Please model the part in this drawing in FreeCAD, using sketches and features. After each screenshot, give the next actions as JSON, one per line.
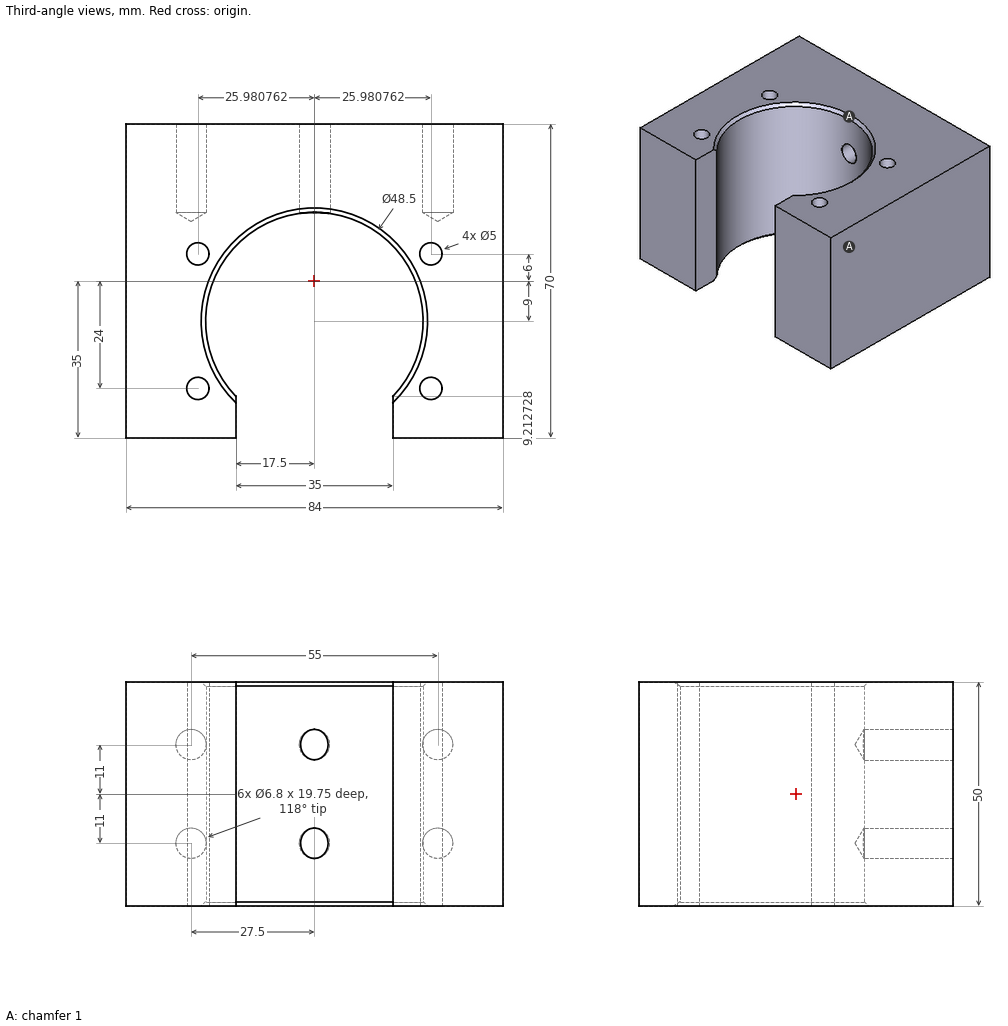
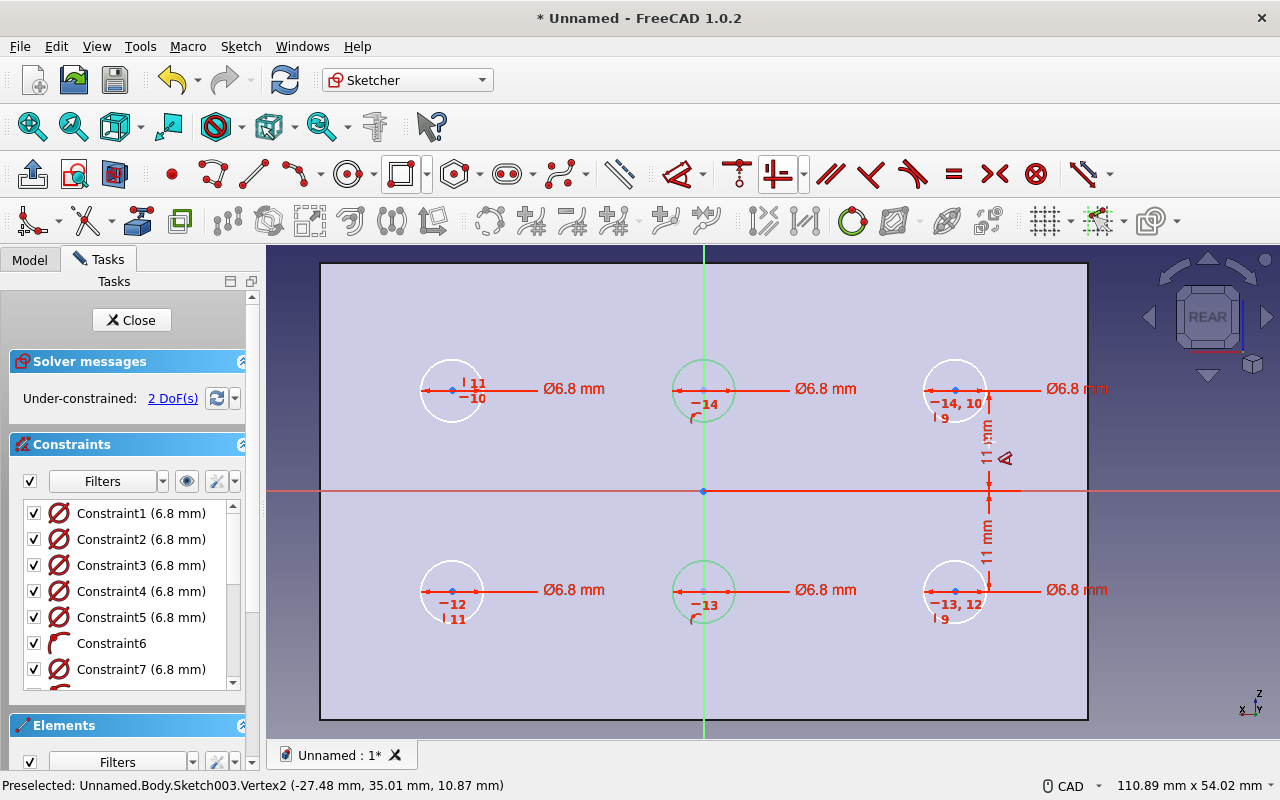
{"action": "left_click", "coordinate": [955, 391]}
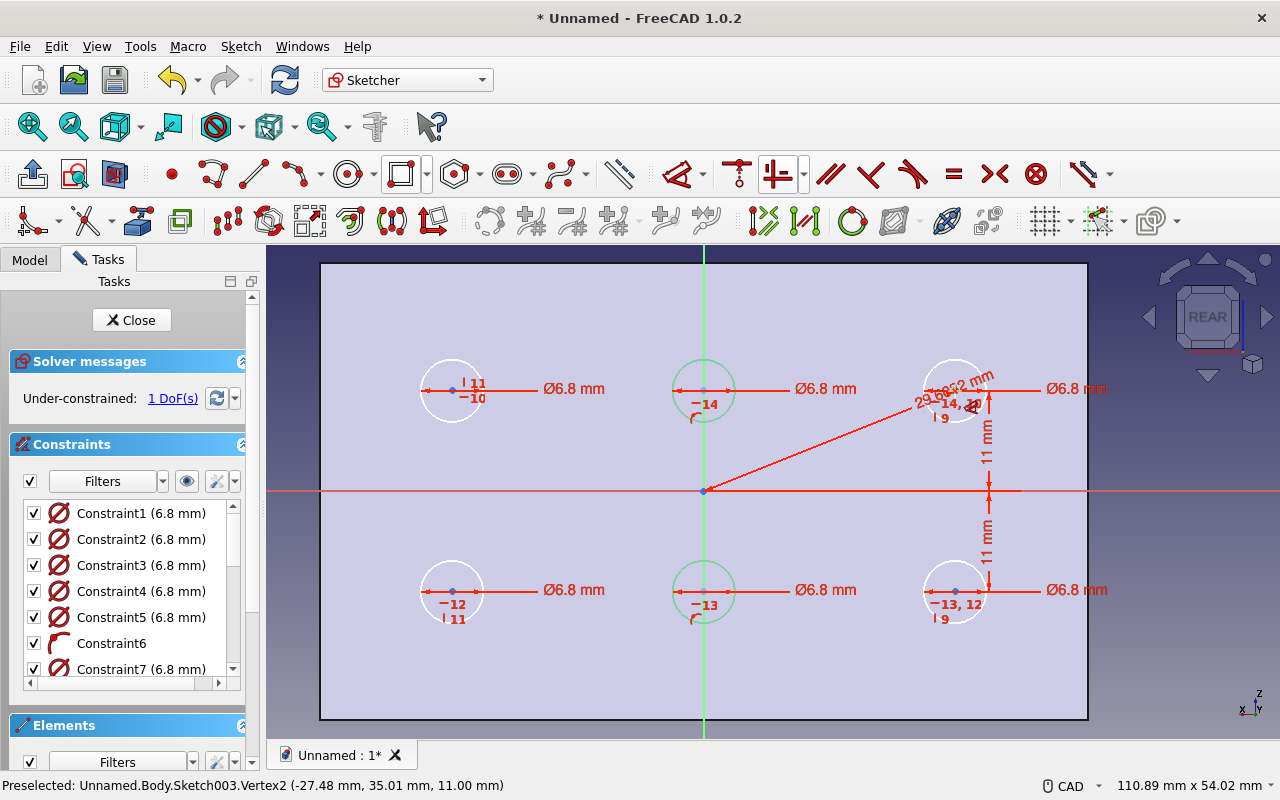
{"action": "left_click", "coordinate": [452, 391]}
{"action": "left_click", "coordinate": [588, 357]}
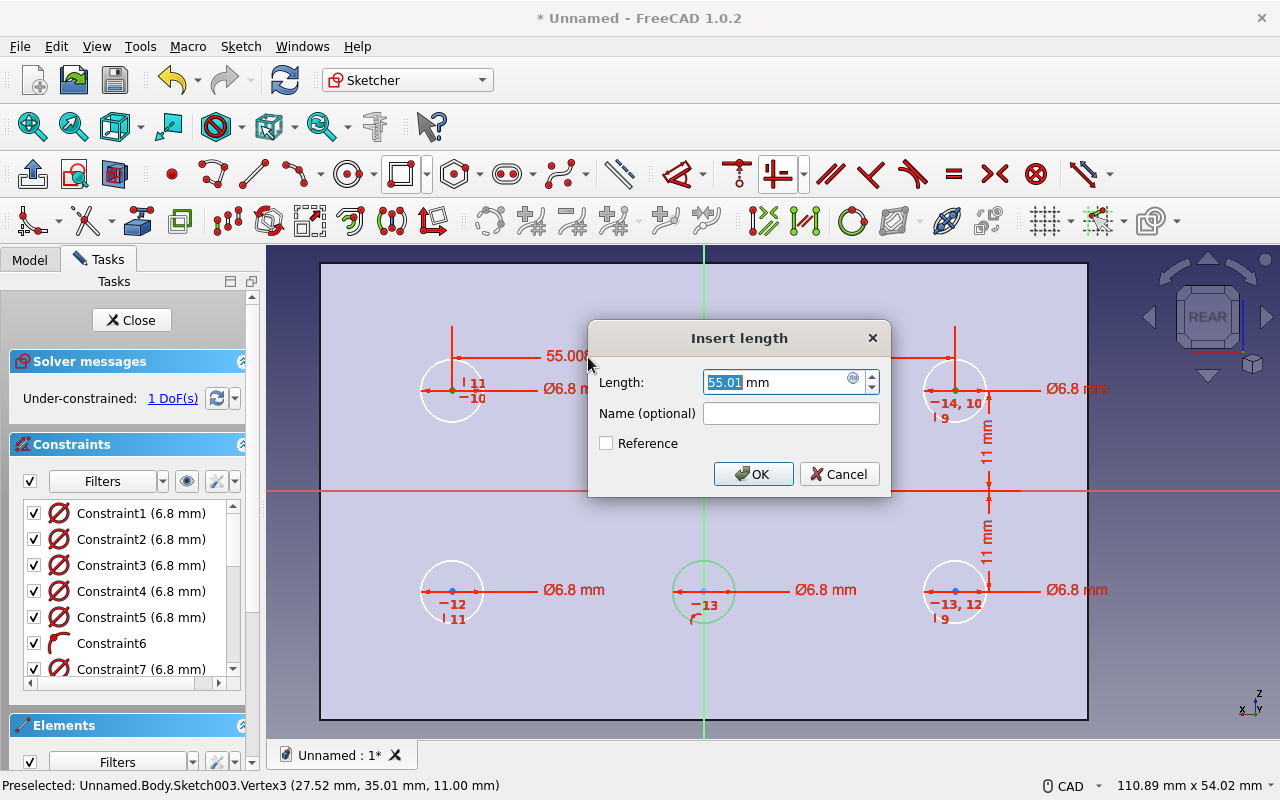
{"action": "type", "text": "55"}
{"action": "key", "text": "Return"}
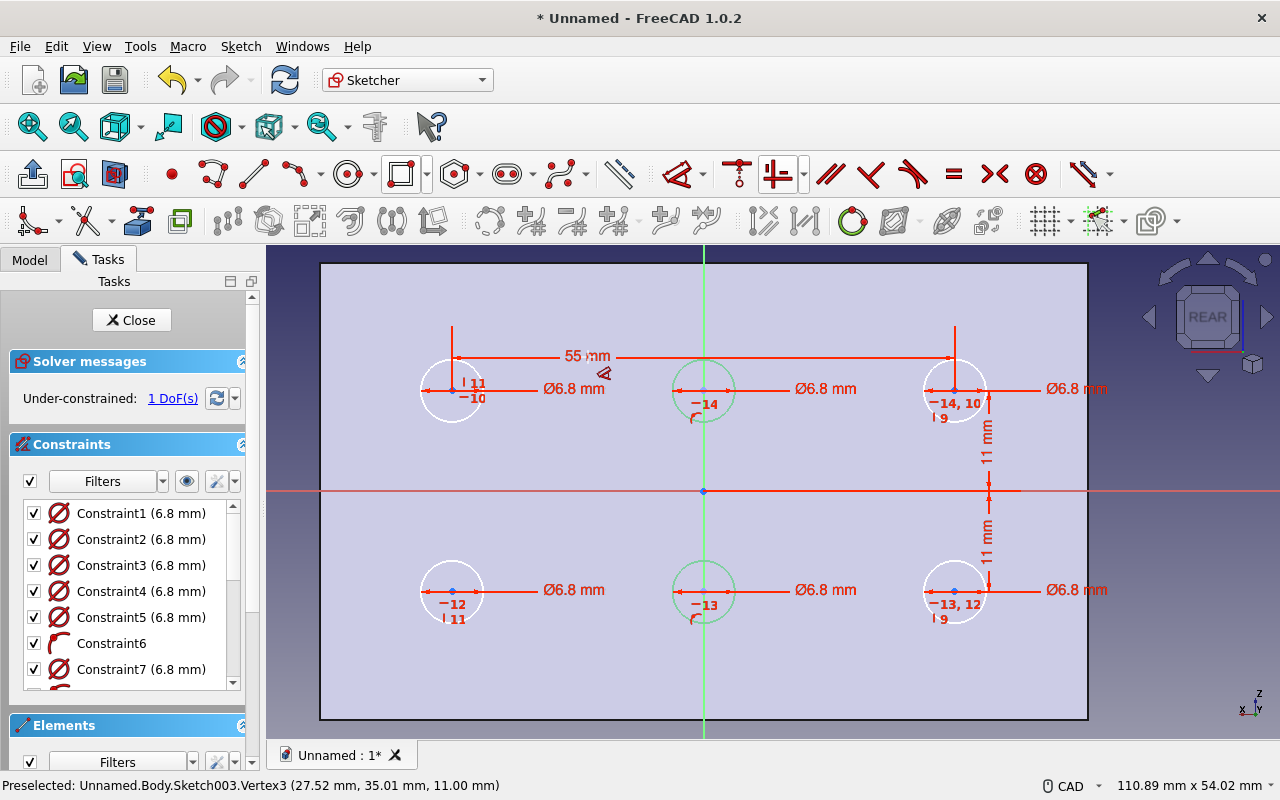
{"action": "left_click", "coordinate": [955, 592]}
{"action": "left_click", "coordinate": [829, 626]}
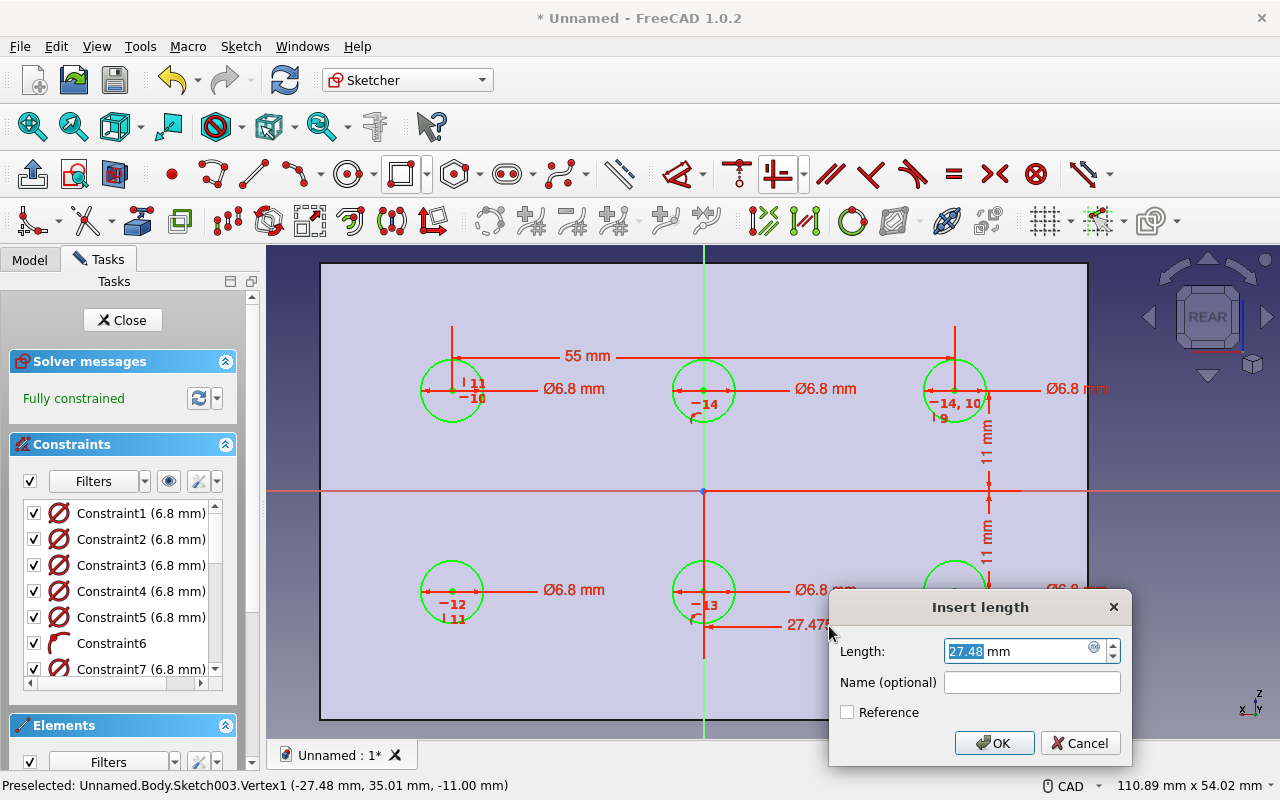
{"action": "type", "text": "27.5"}
{"action": "key", "text": "Return"}
{"action": "key", "text": "Escape"}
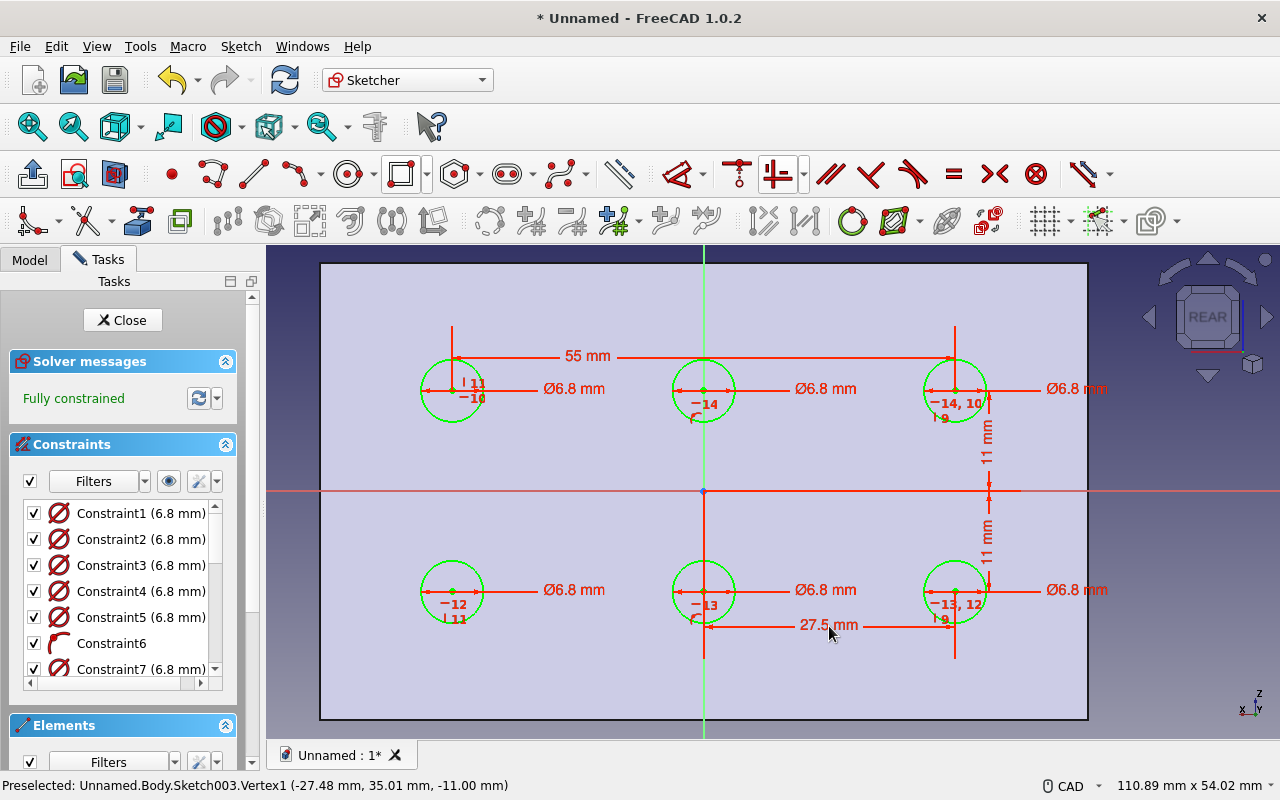
{"action": "left_click", "coordinate": [123, 320]}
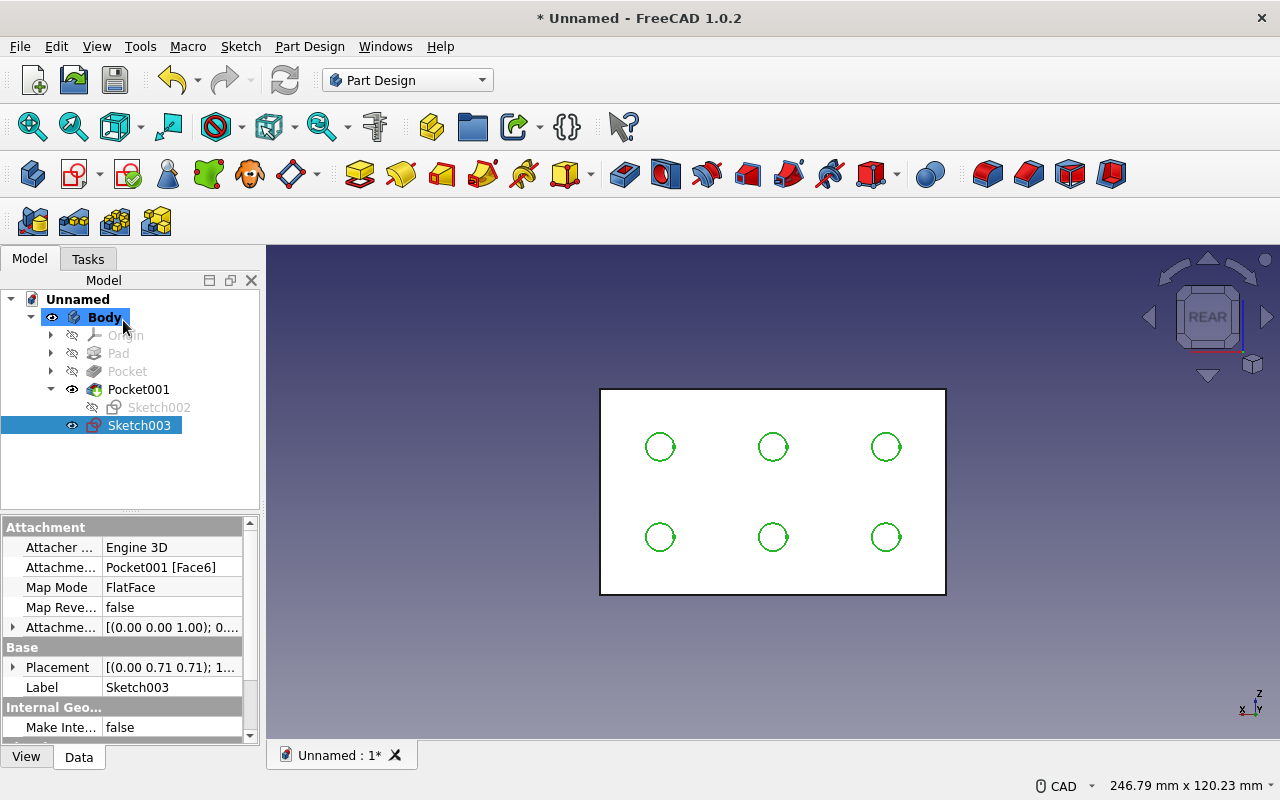
{"action": "left_click", "coordinate": [666, 174]}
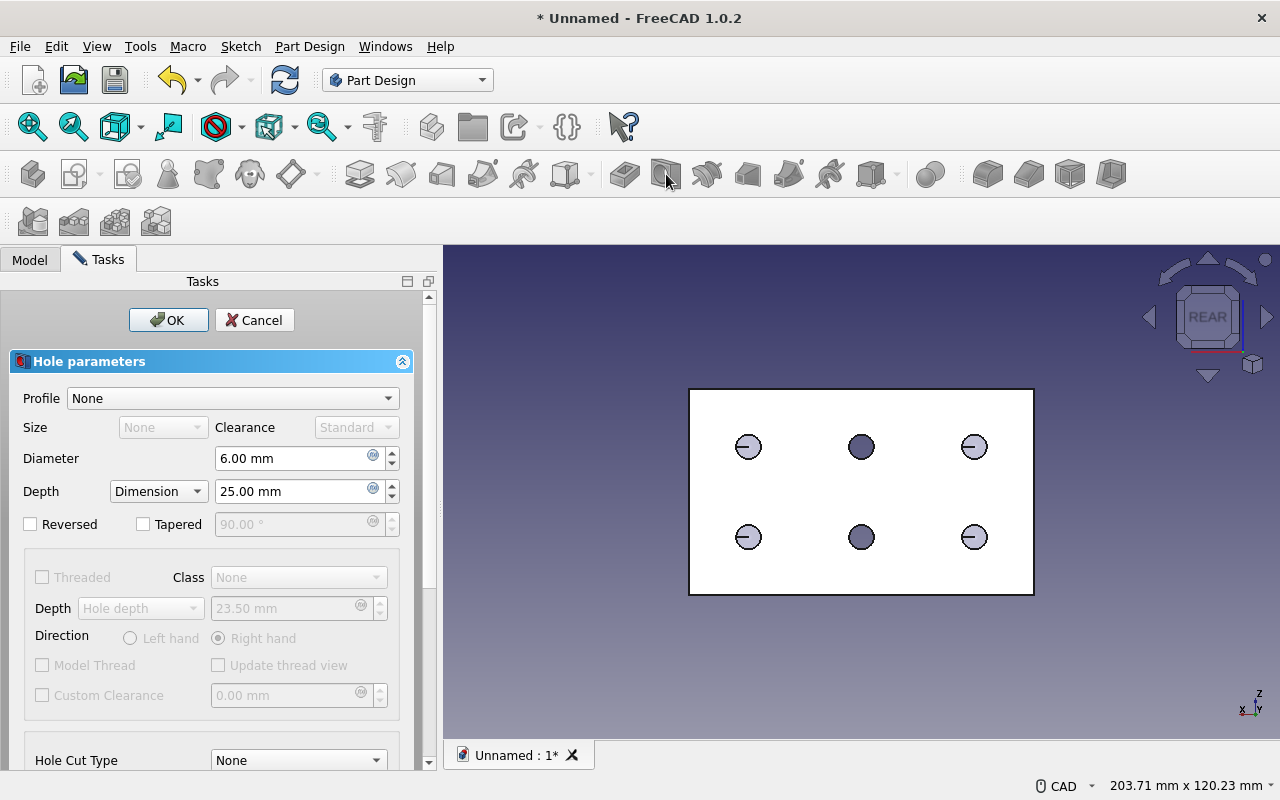
{"action": "triple_click", "coordinate": [300, 458]}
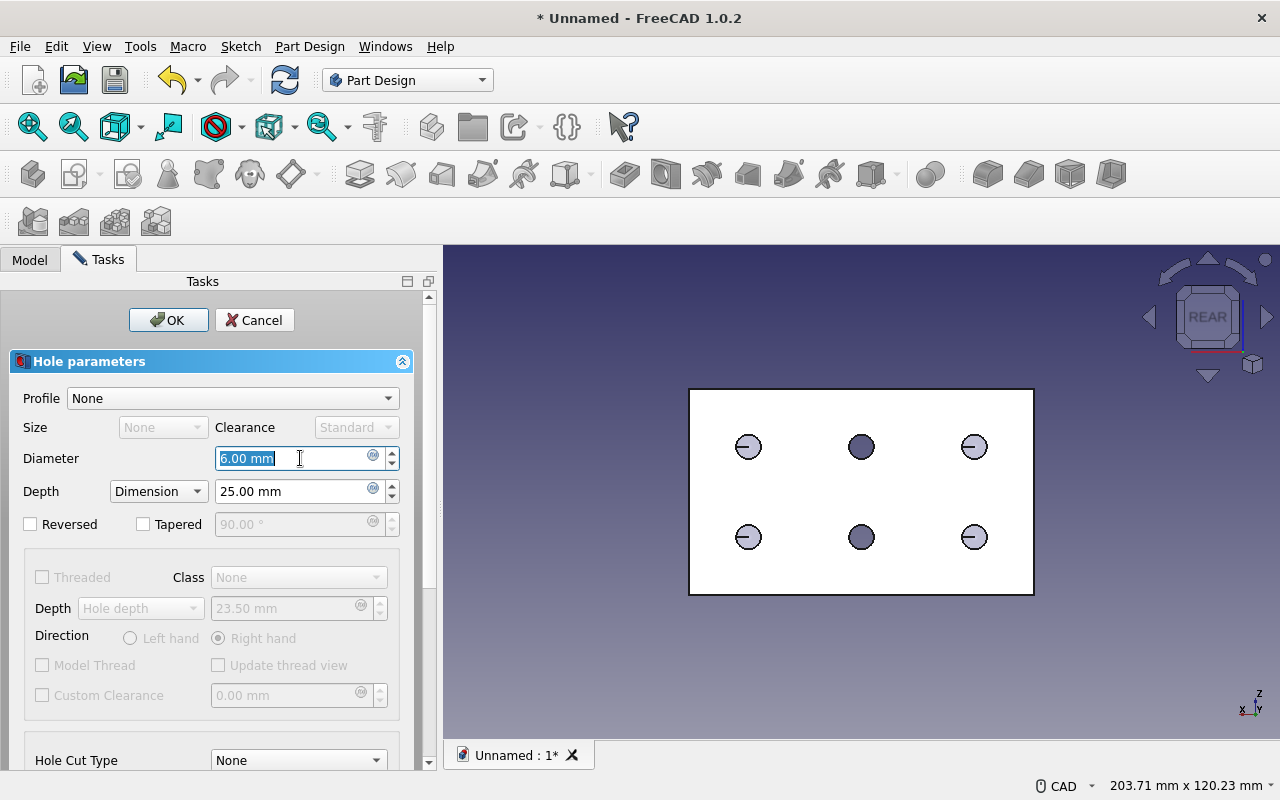
{"action": "type", "text": "6.8"}
{"action": "key", "text": "Tab"}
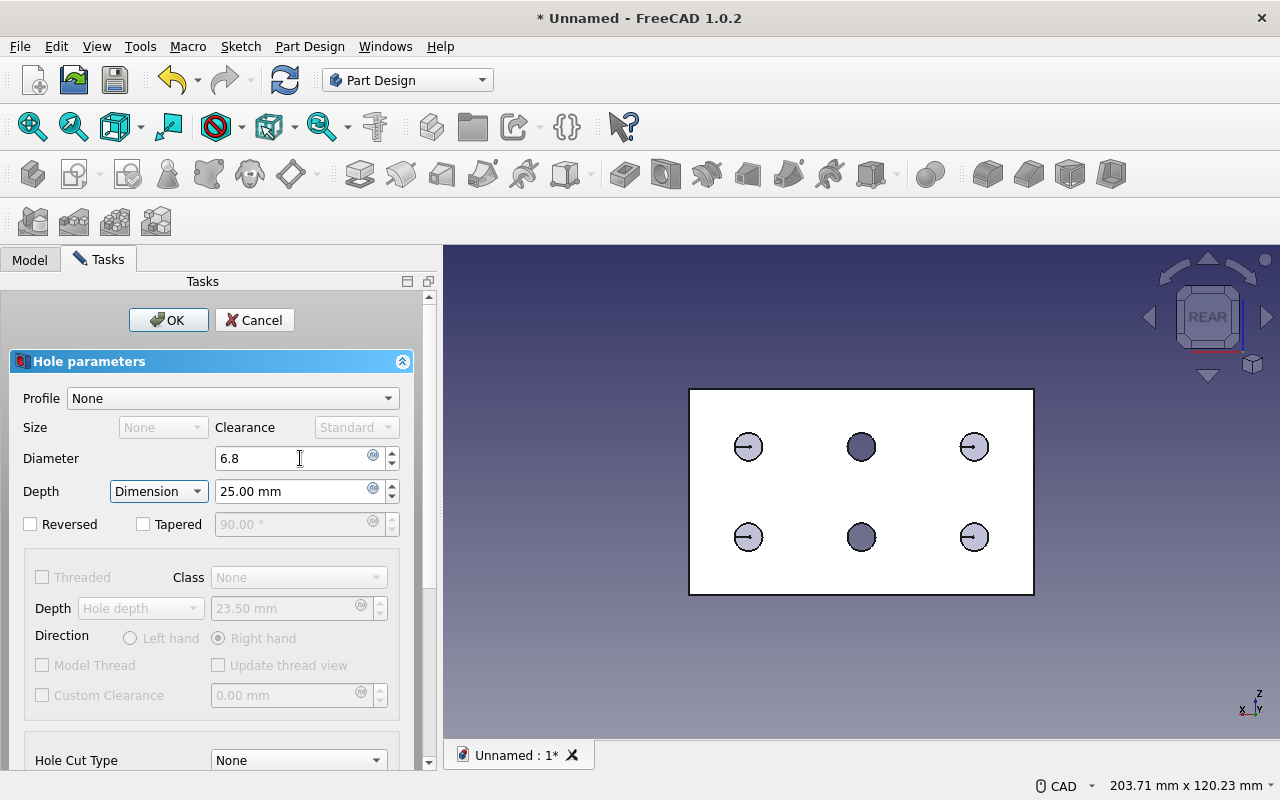
{"action": "triple_click", "coordinate": [300, 492]}